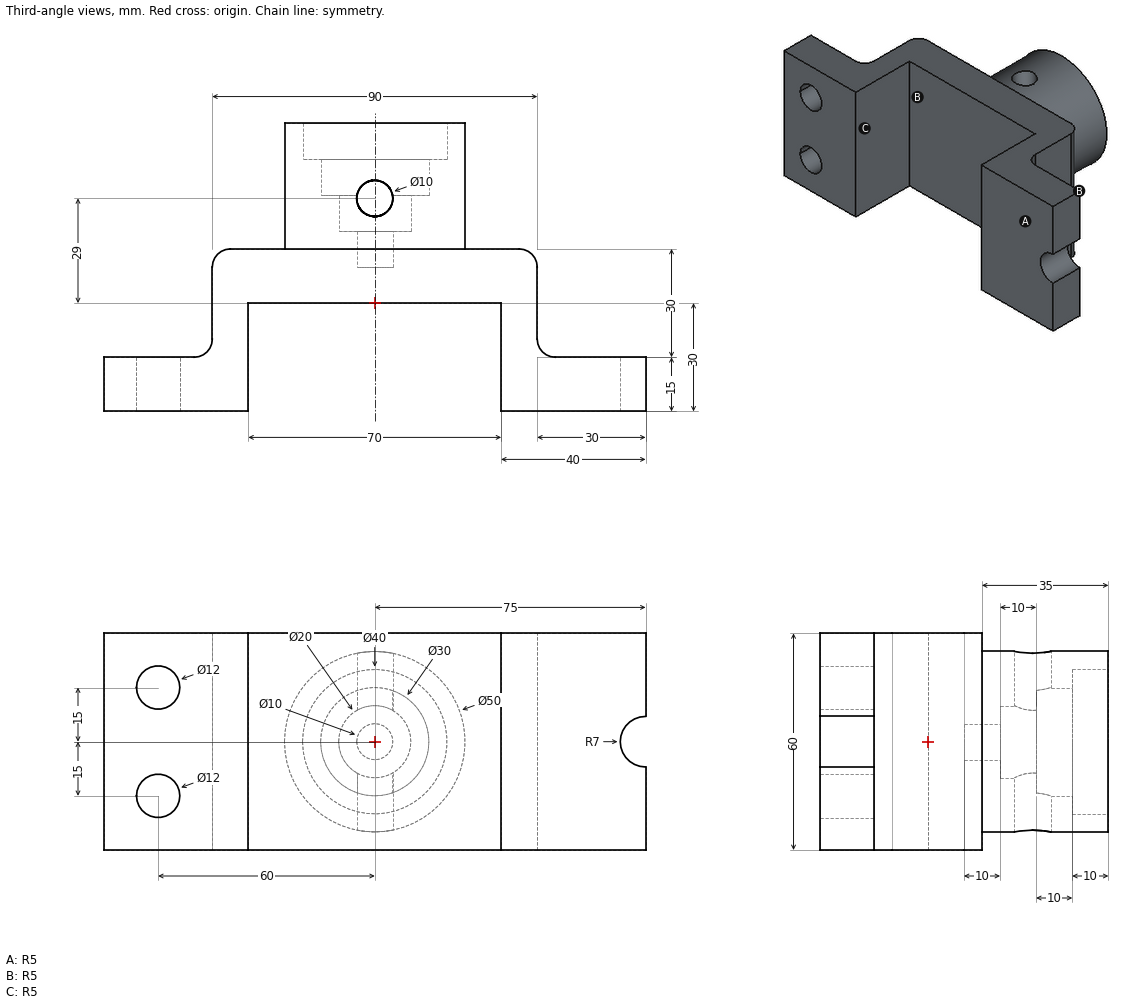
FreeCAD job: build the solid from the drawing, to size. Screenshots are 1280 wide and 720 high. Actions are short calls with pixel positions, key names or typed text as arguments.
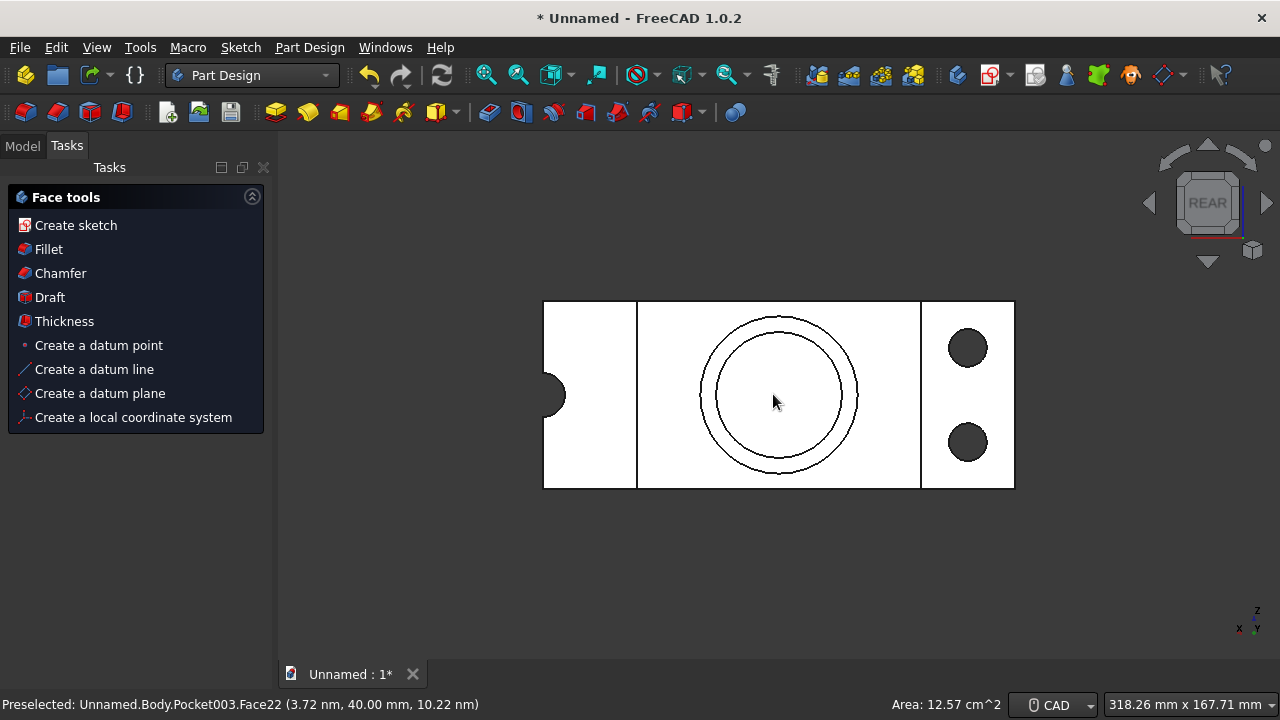
click(990, 76)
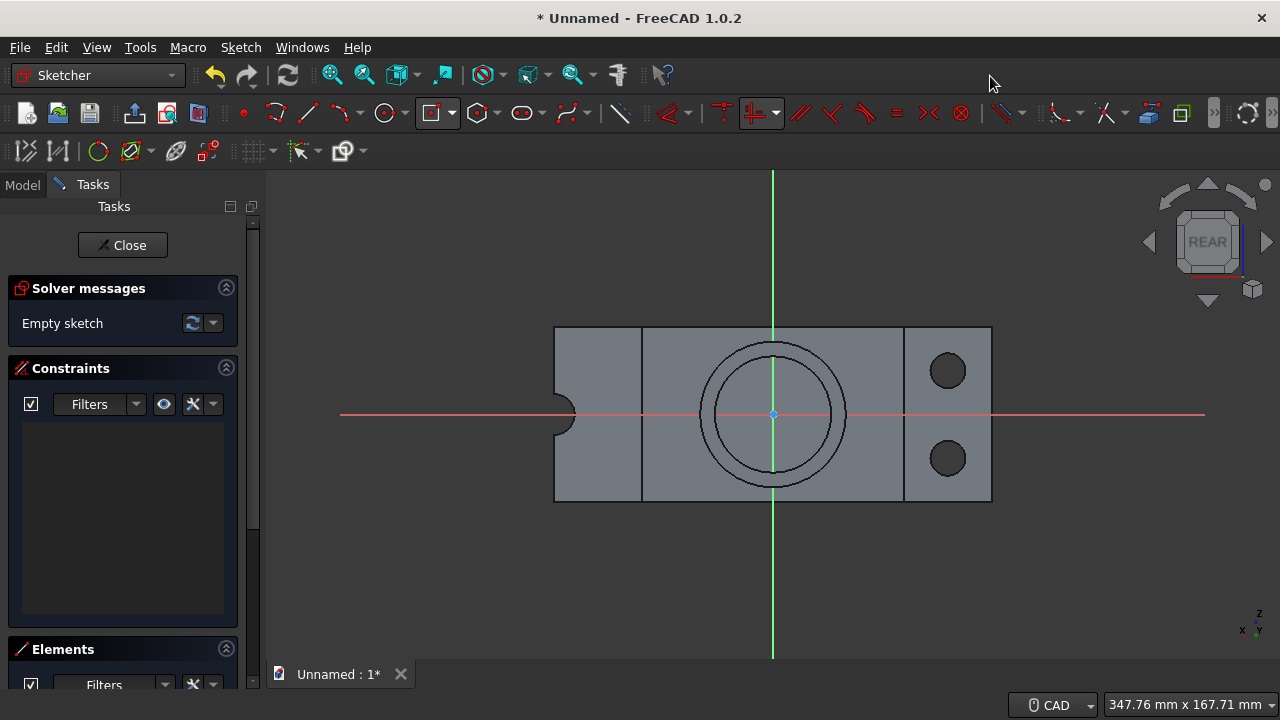
scroll(803, 415, up, 6)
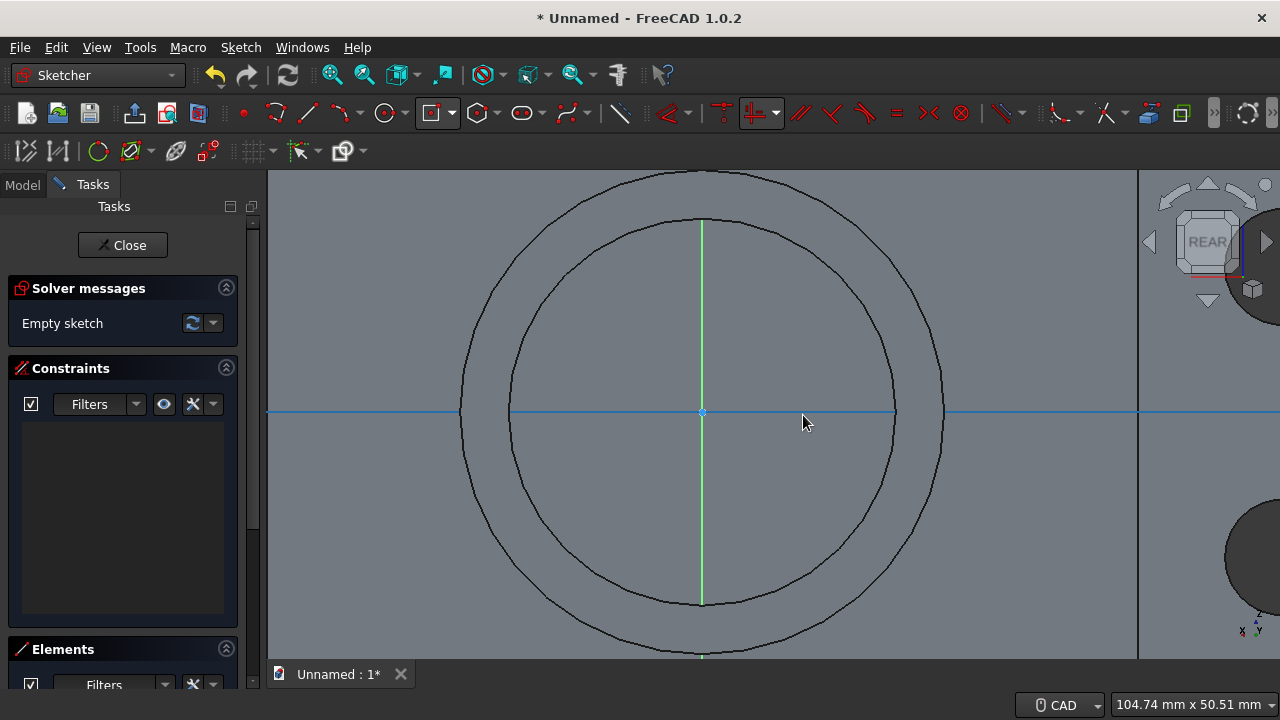
click(386, 114)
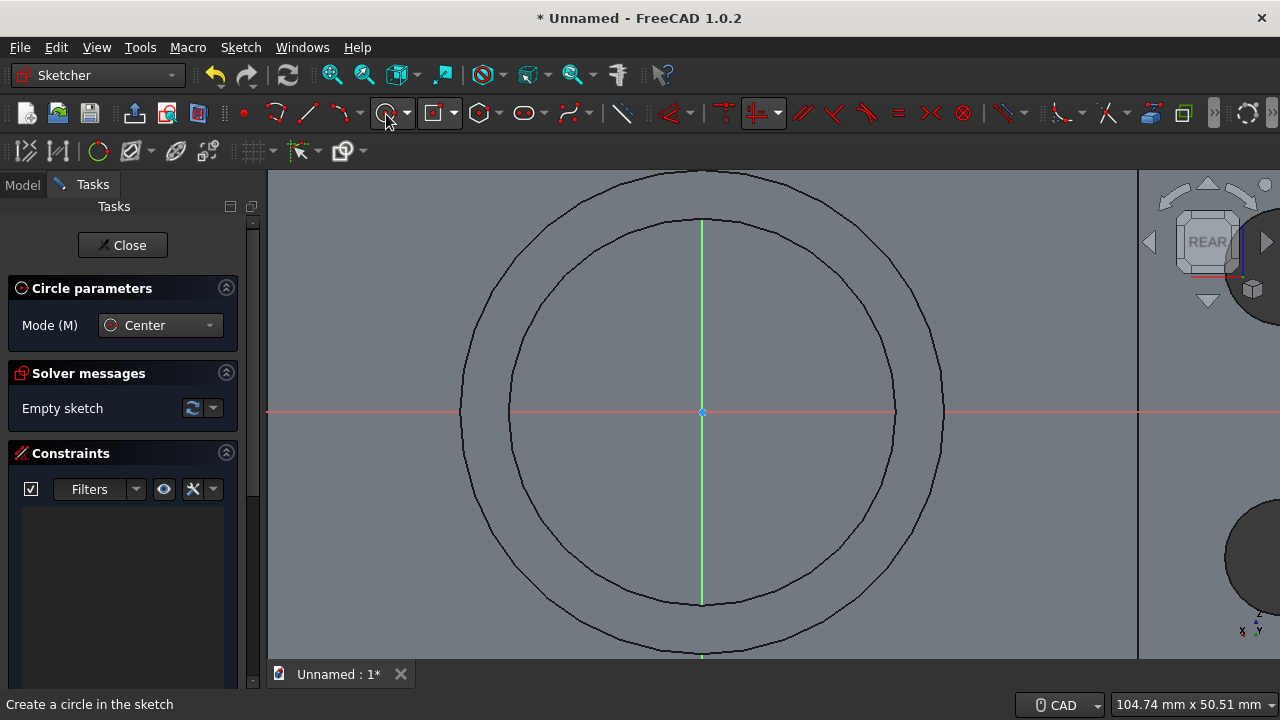
click(702, 412)
click(805, 309)
key(Escape)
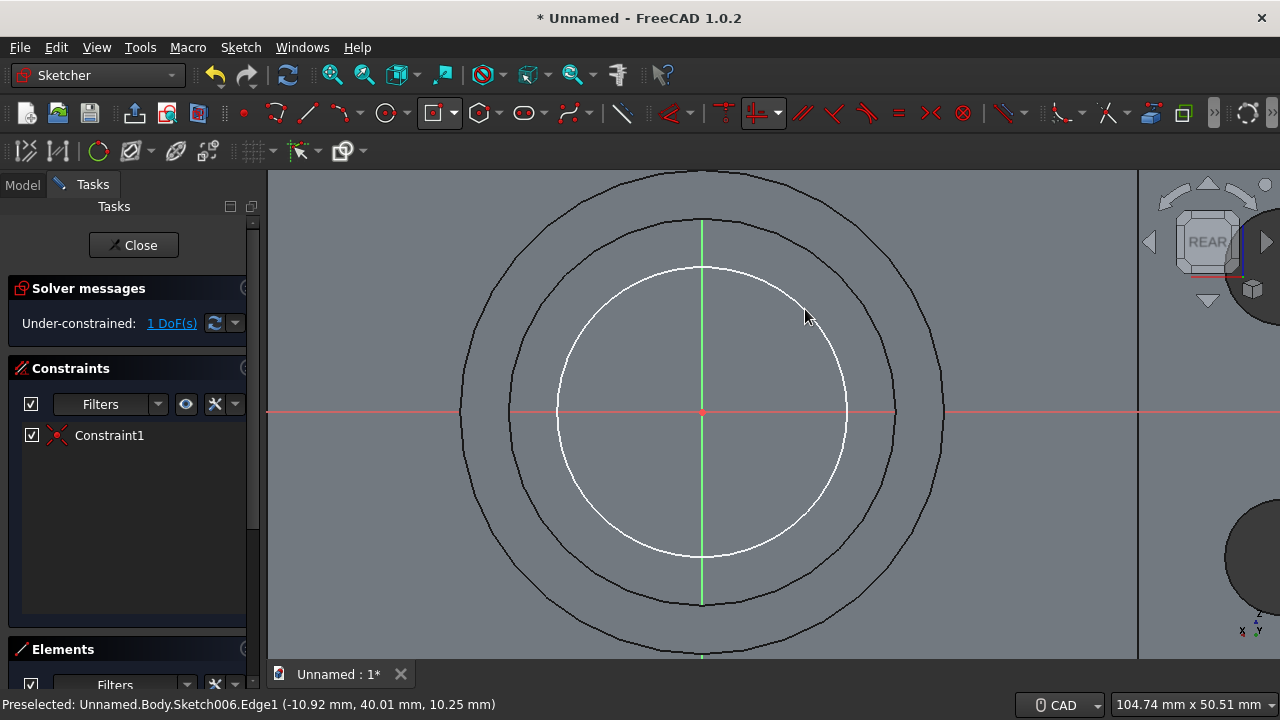
click(670, 114)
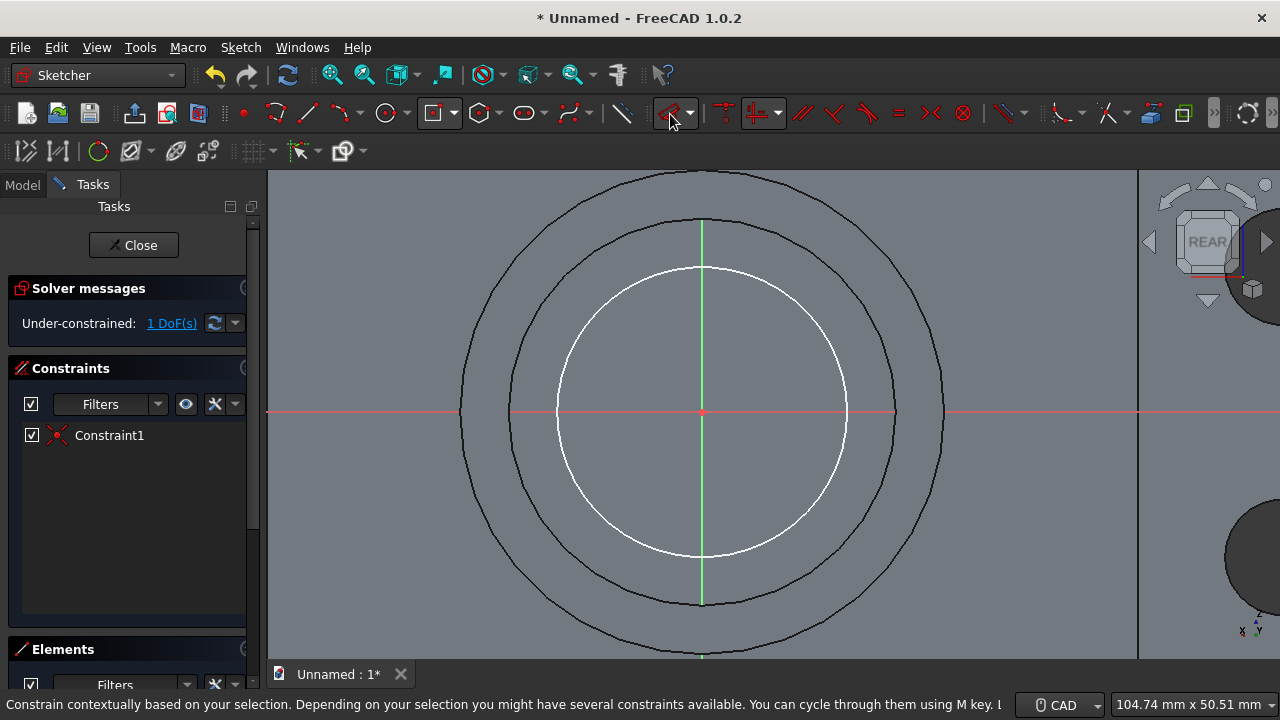
click(804, 309)
click(826, 286)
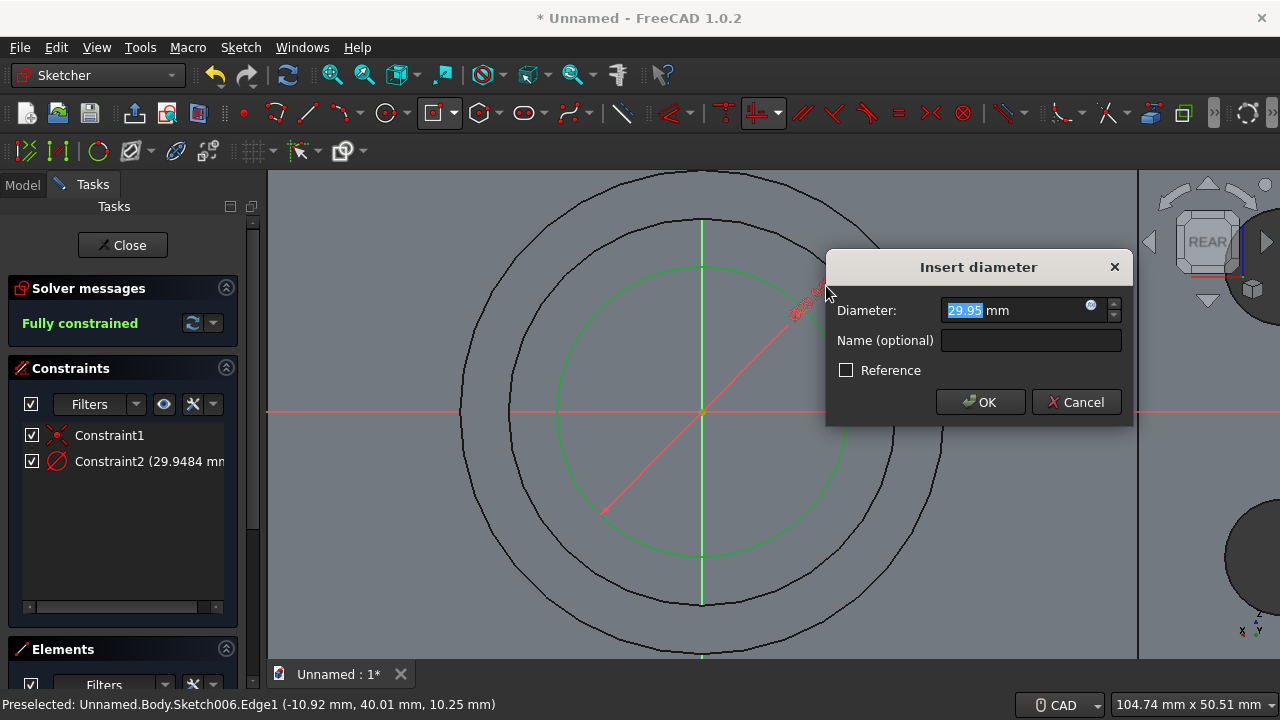
text(30)
key(Return)
key(Escape)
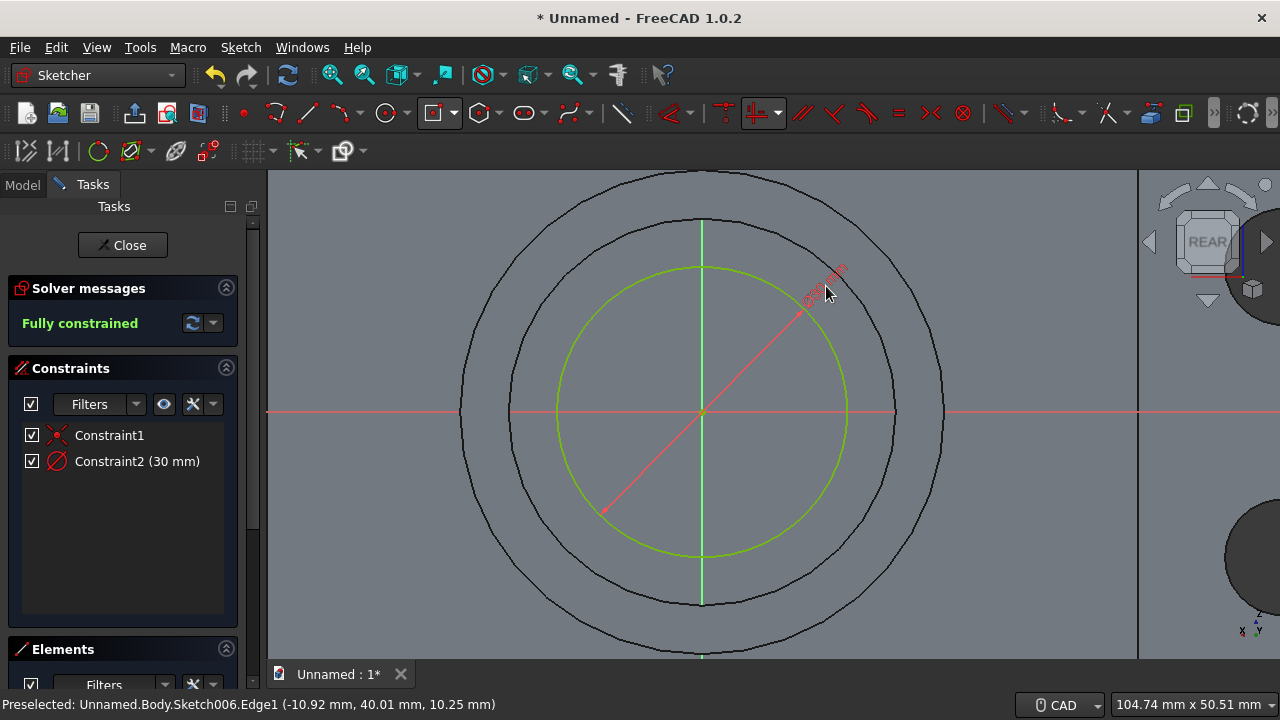
click(123, 245)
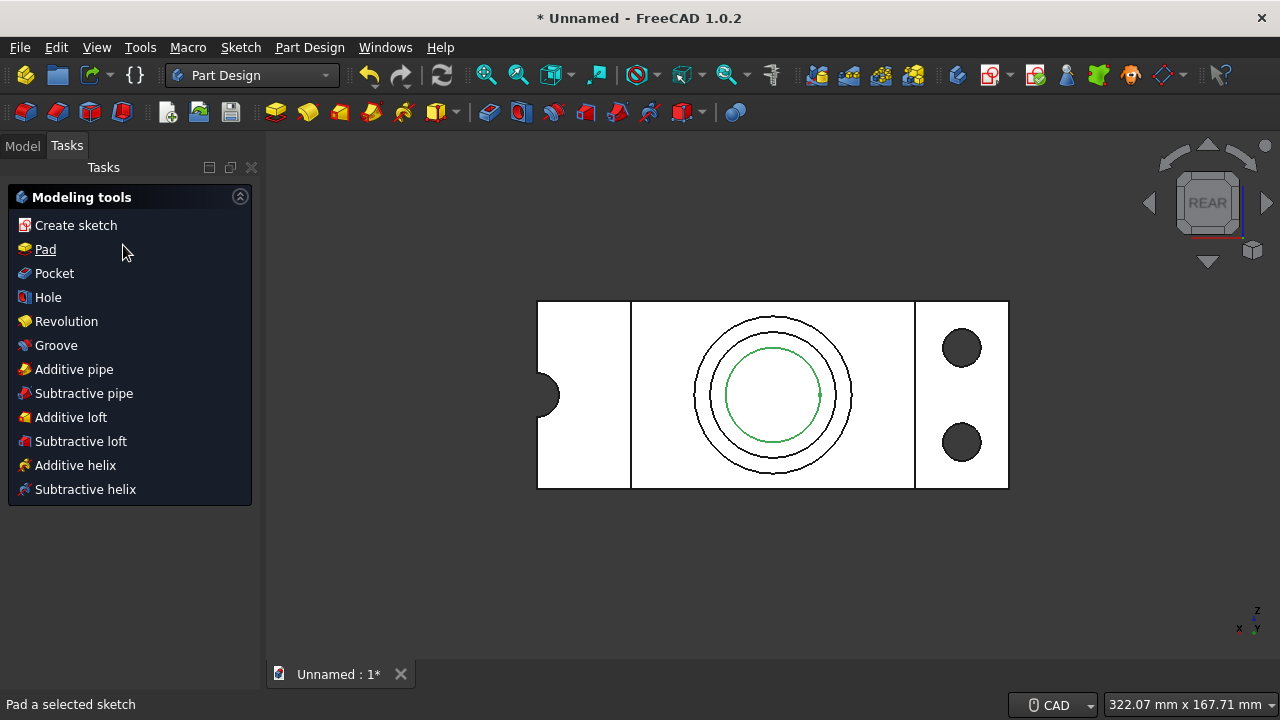
click(490, 112)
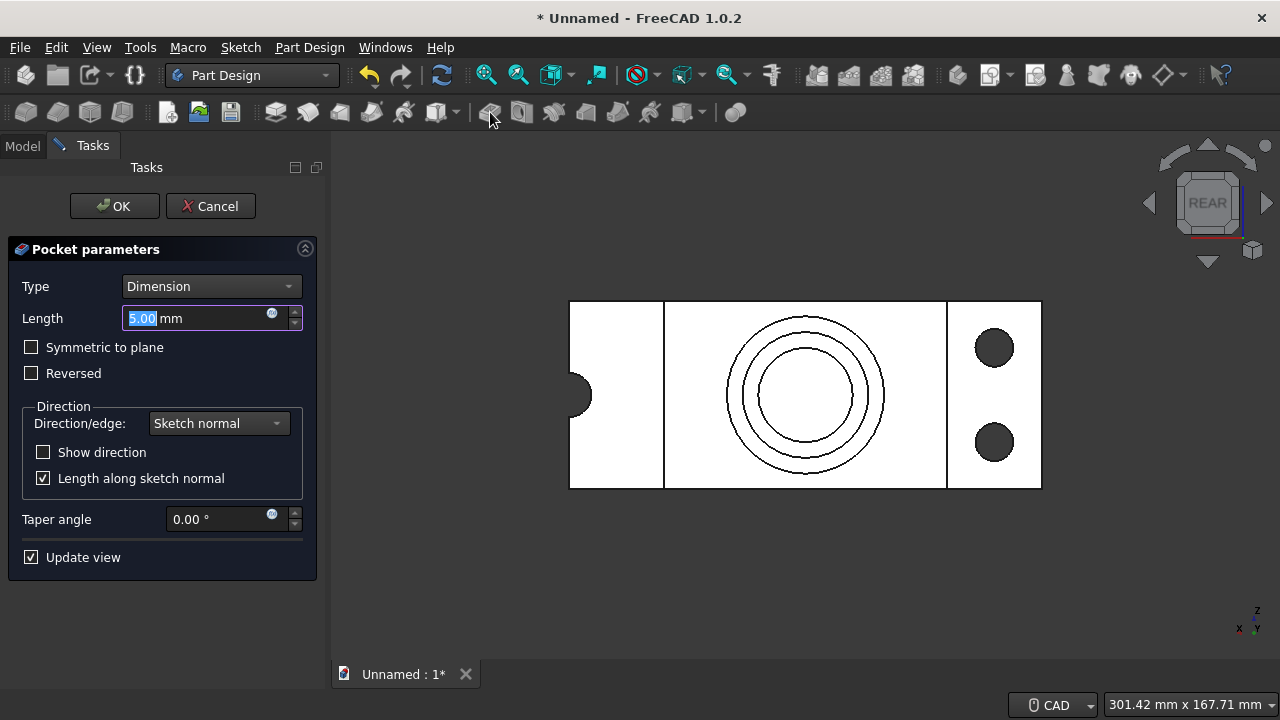
text(10)
key(Tab)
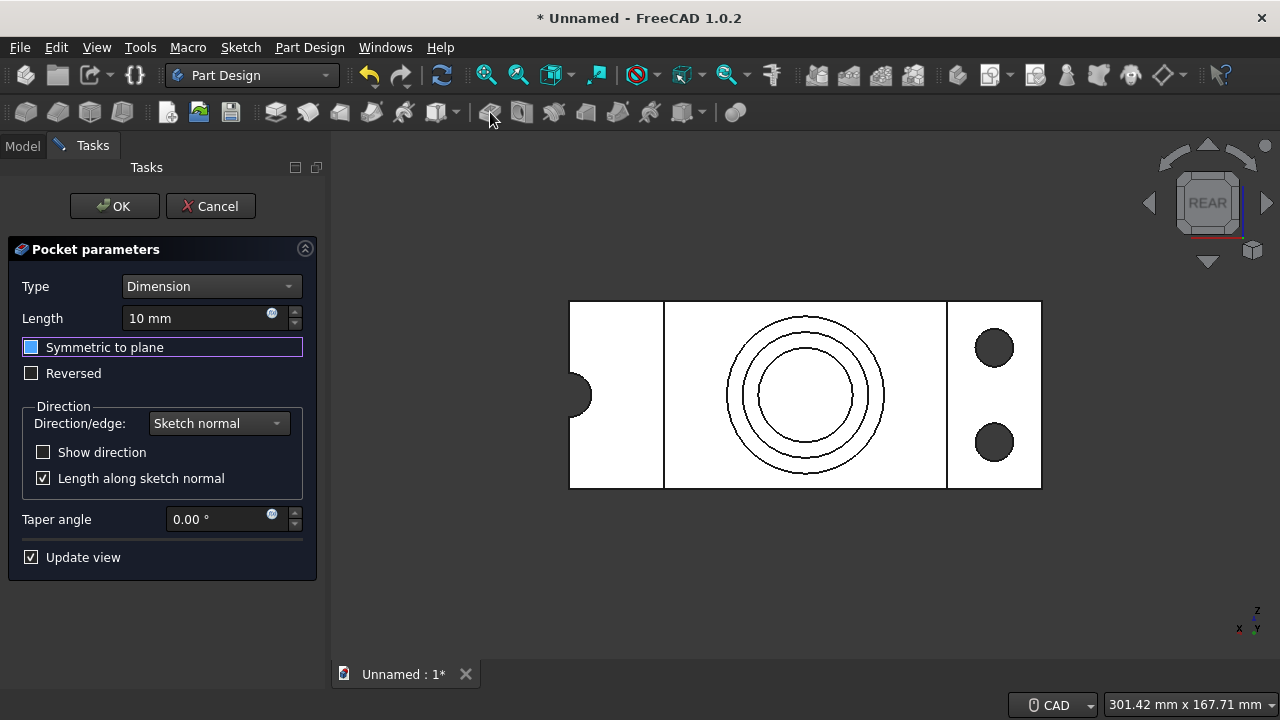
click(115, 206)